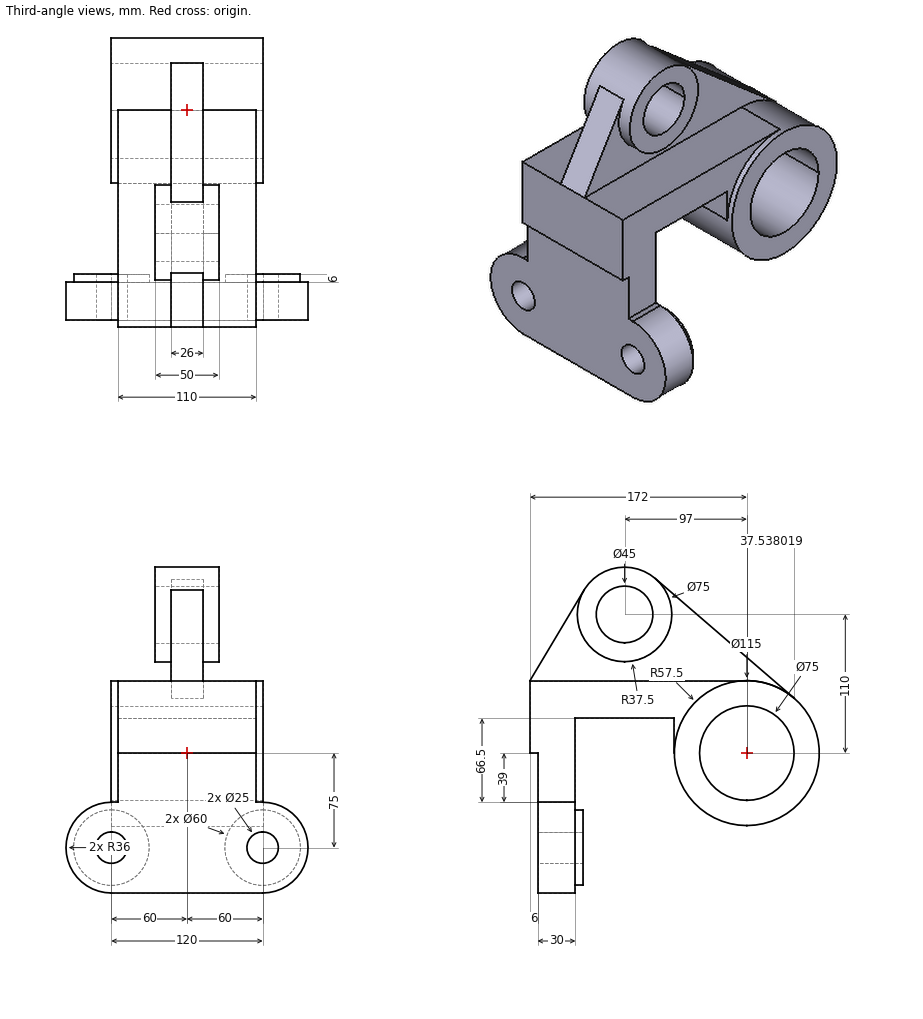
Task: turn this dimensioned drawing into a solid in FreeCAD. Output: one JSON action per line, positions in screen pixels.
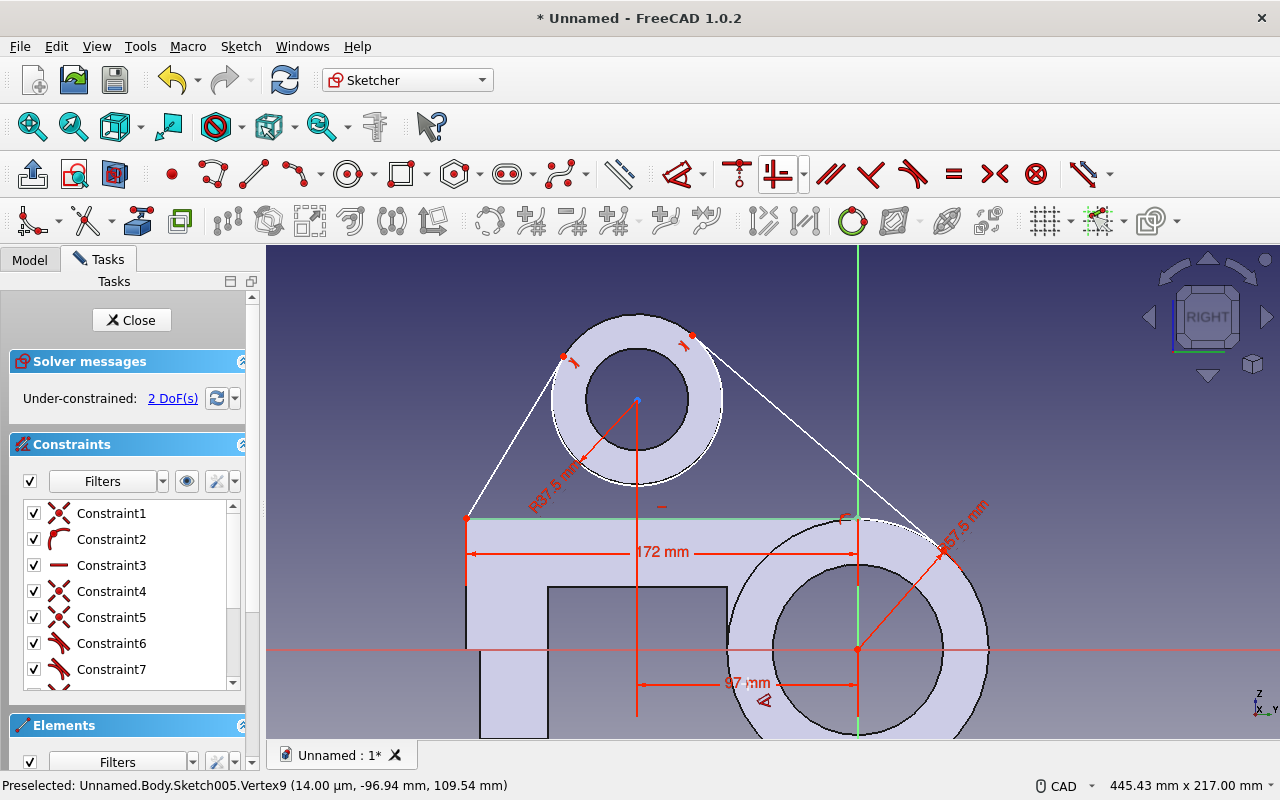
{"action": "left_click", "coordinate": [637, 400]}
{"action": "left_click", "coordinate": [892, 468]}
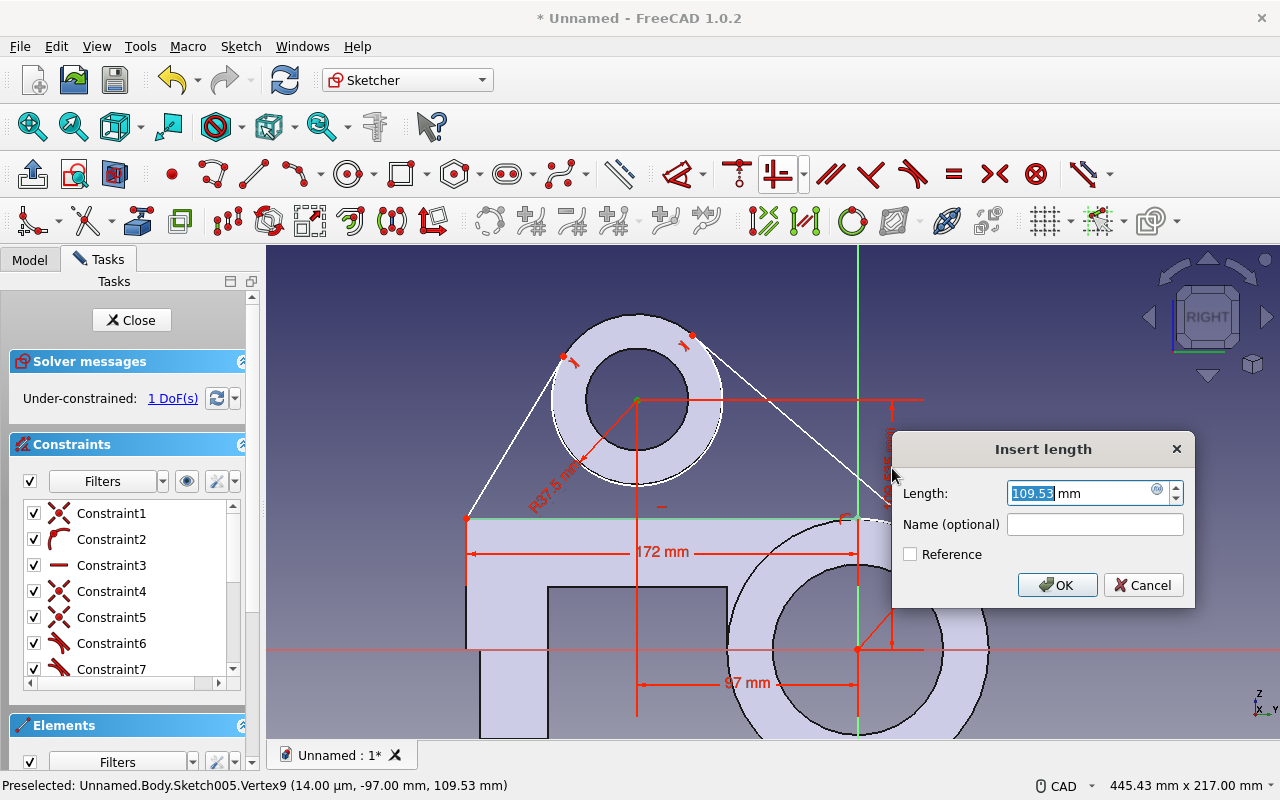
{"action": "type", "text": "110"}
{"action": "key", "text": "Return"}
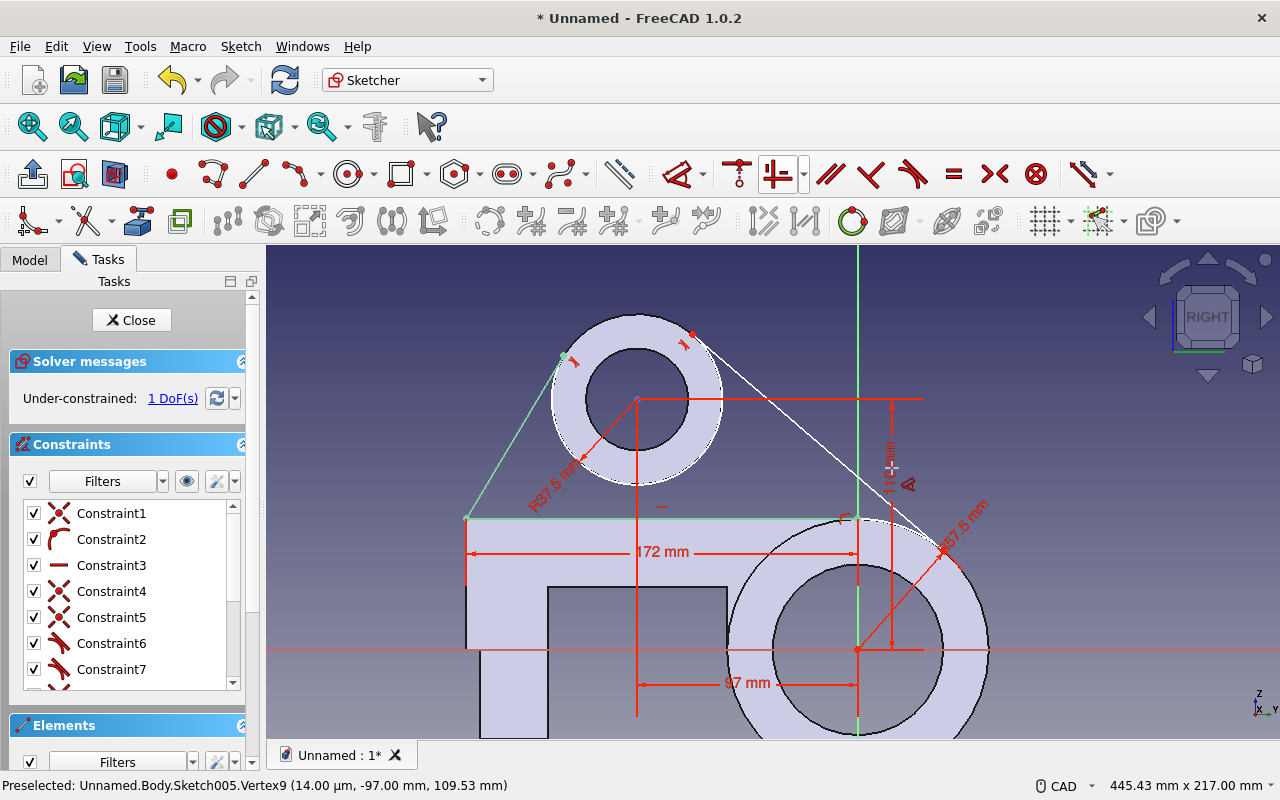
{"action": "left_click", "coordinate": [943, 550]}
{"action": "left_click", "coordinate": [901, 684]}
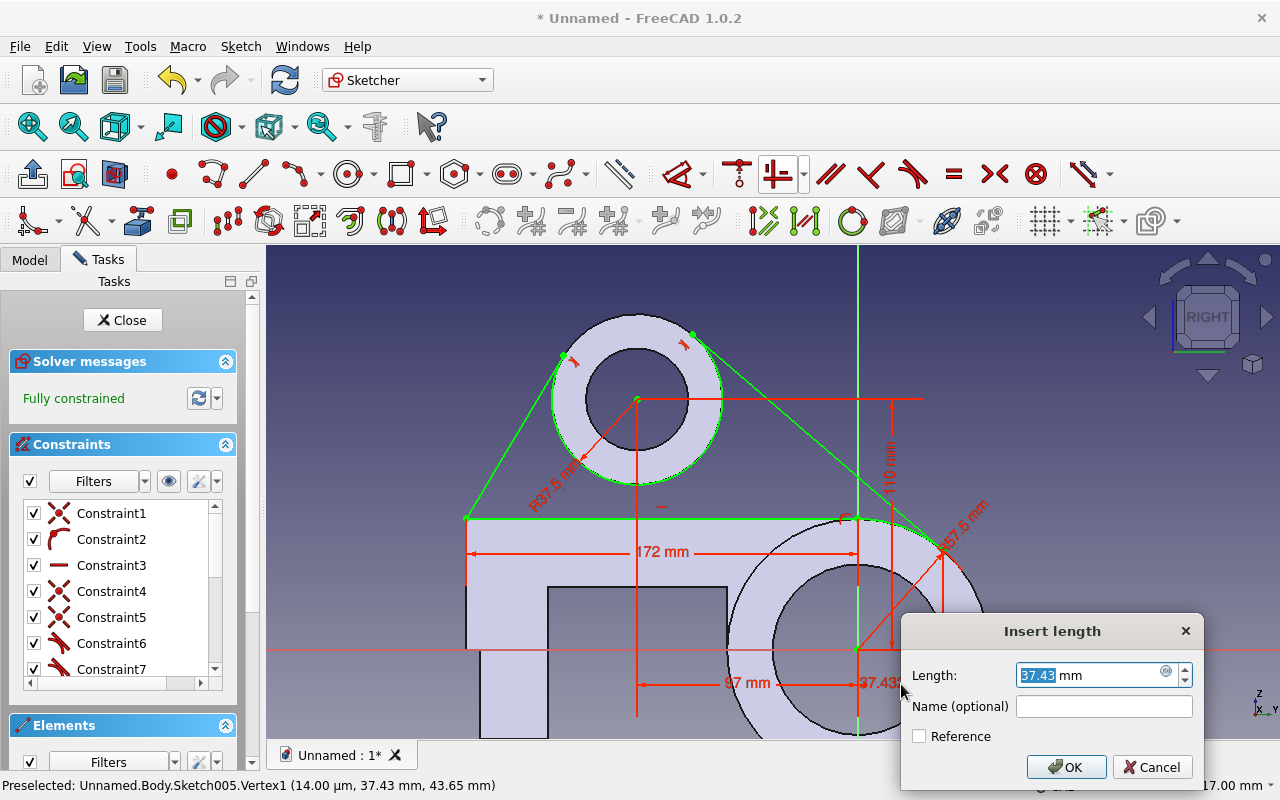
{"action": "type", "text": "37.538019"}
{"action": "key", "text": "Return"}
{"action": "key", "text": "Escape"}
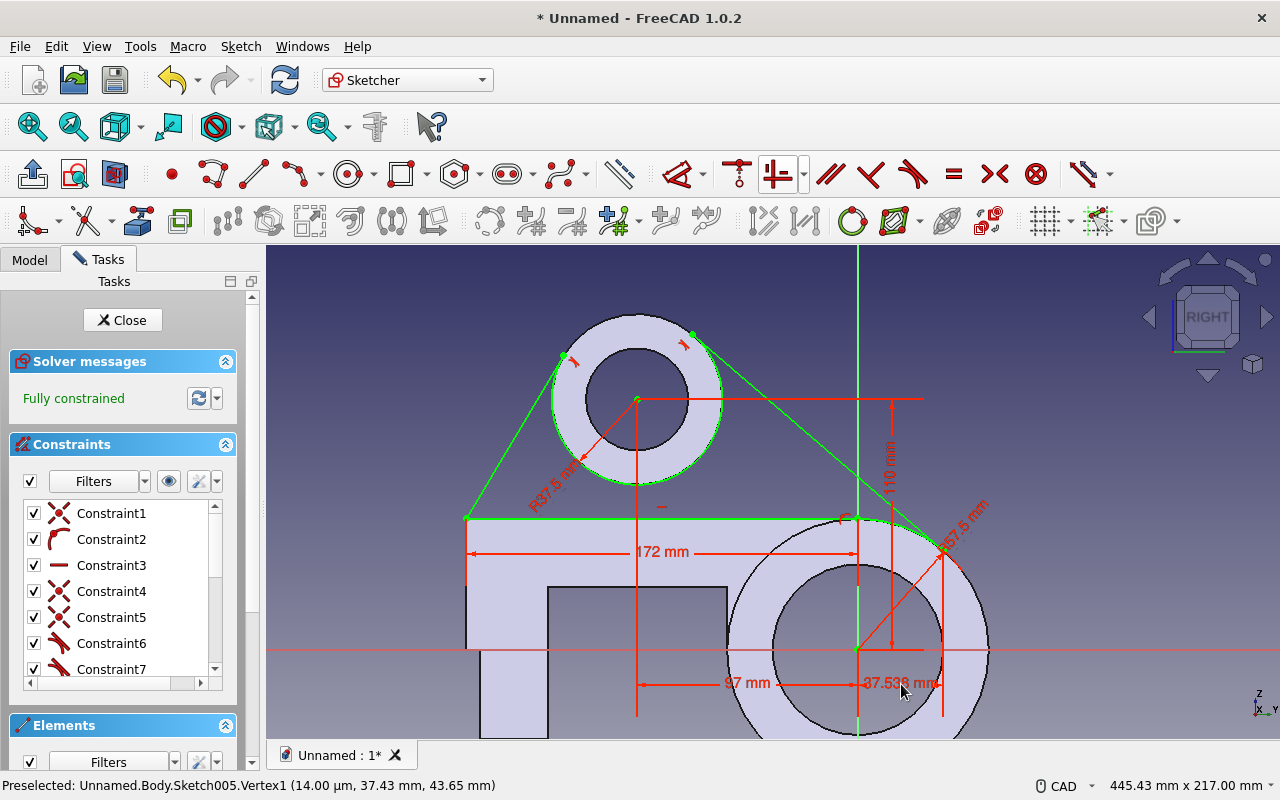
{"action": "left_click", "coordinate": [123, 320]}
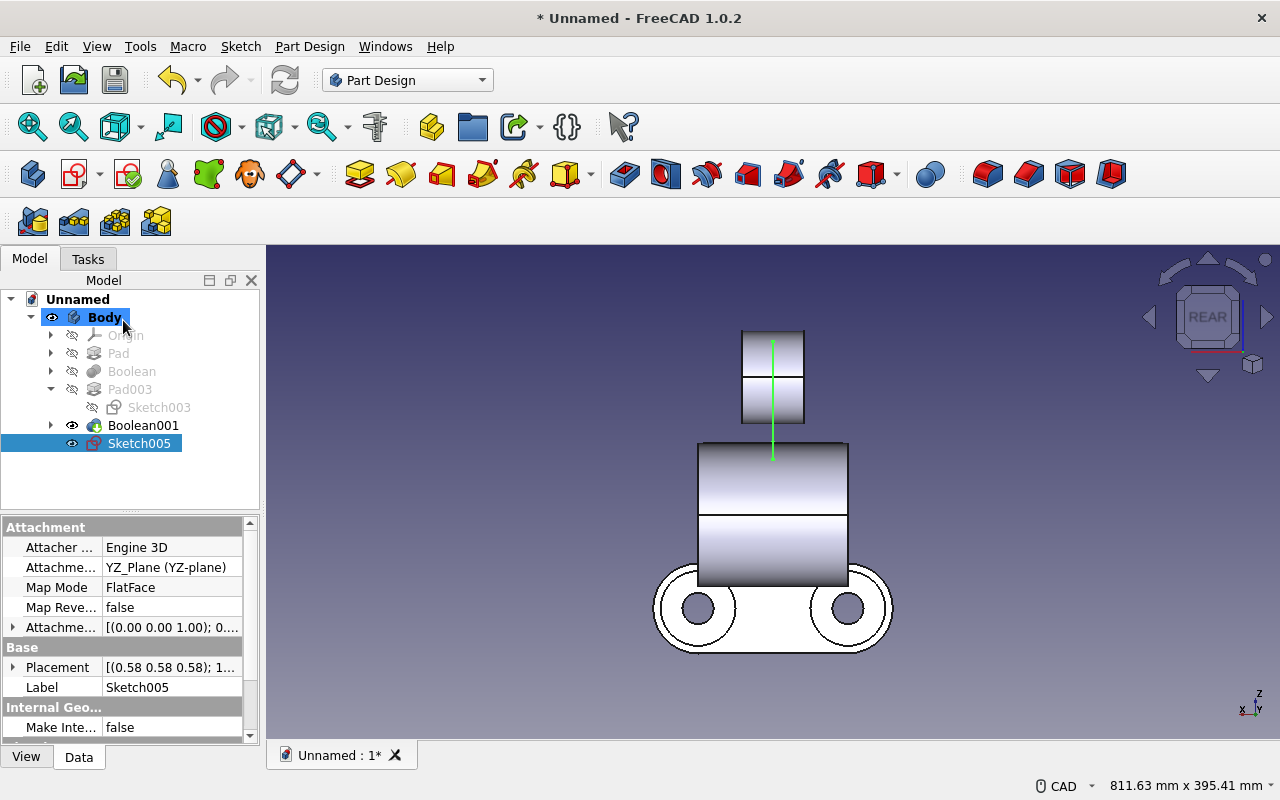
{"action": "left_click", "coordinate": [360, 174]}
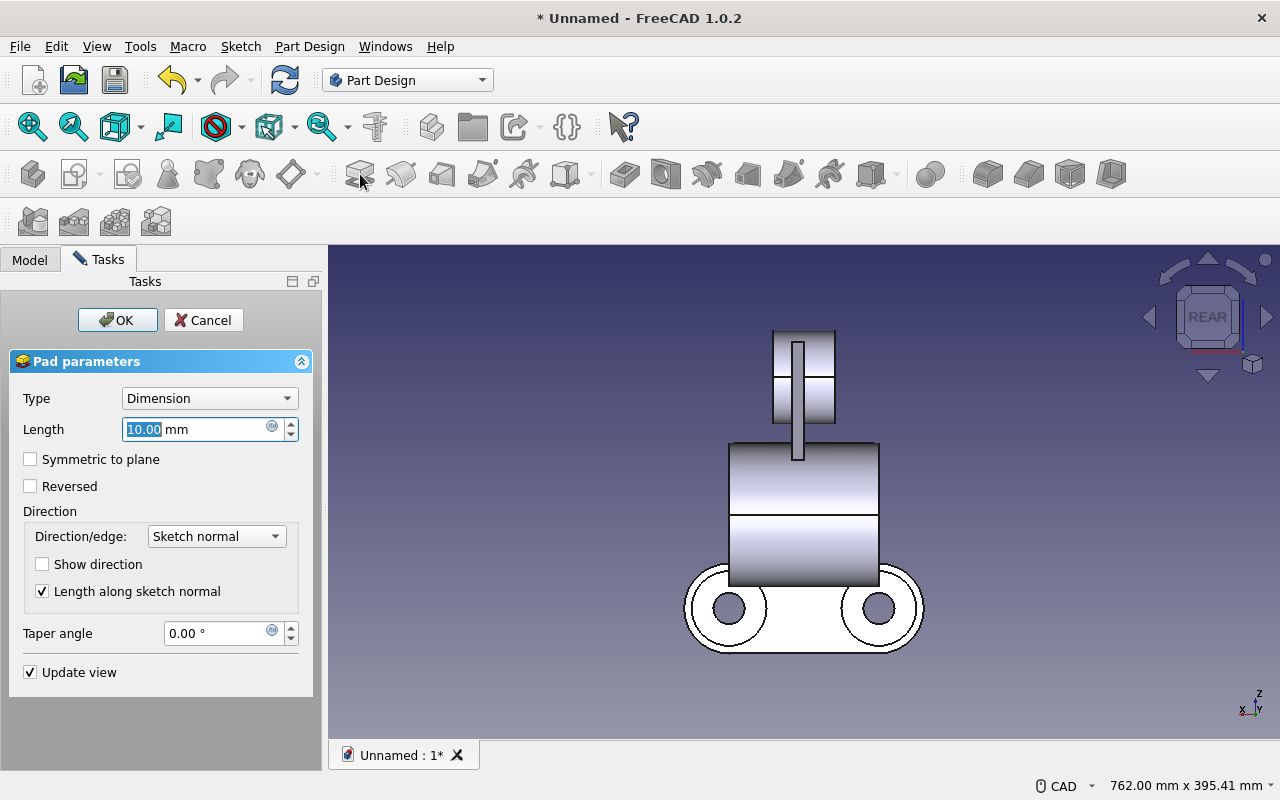
{"action": "type", "text": "26"}
{"action": "key", "text": "Tab"}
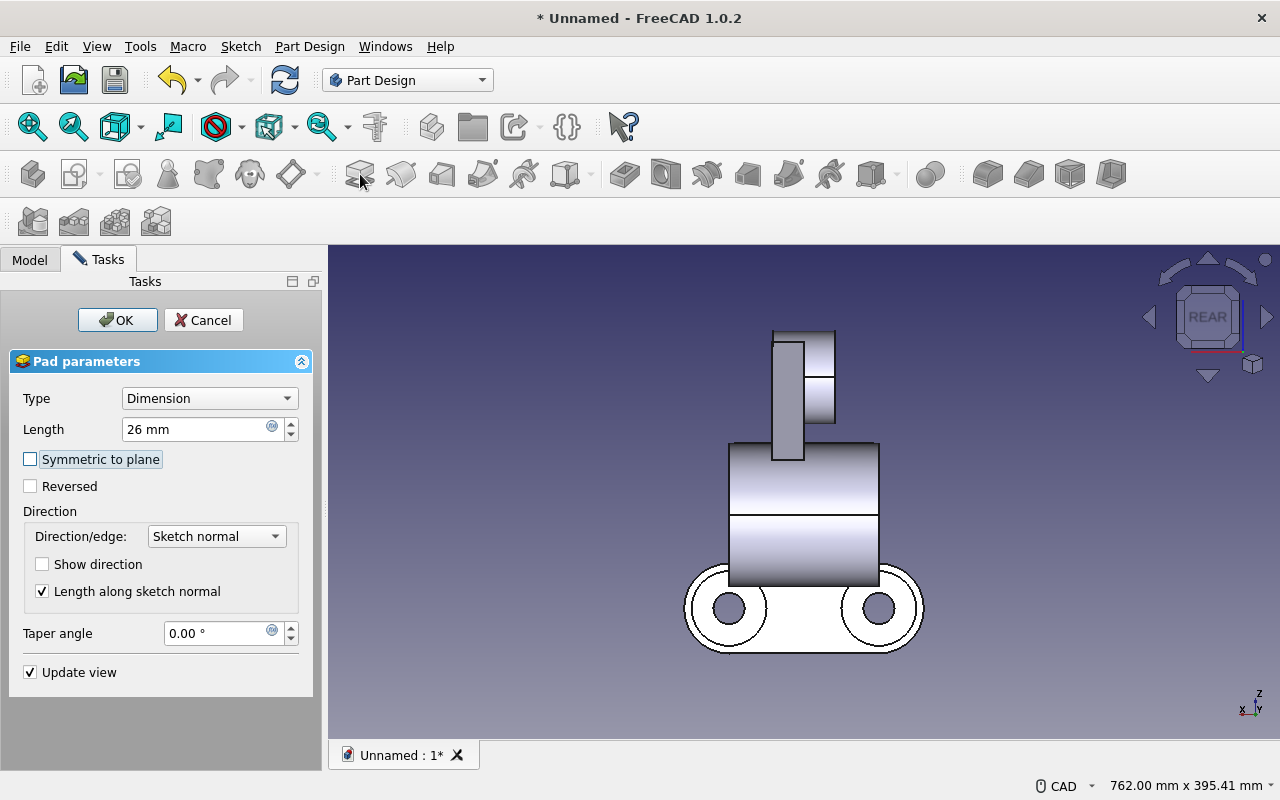
{"action": "left_click", "coordinate": [31, 459]}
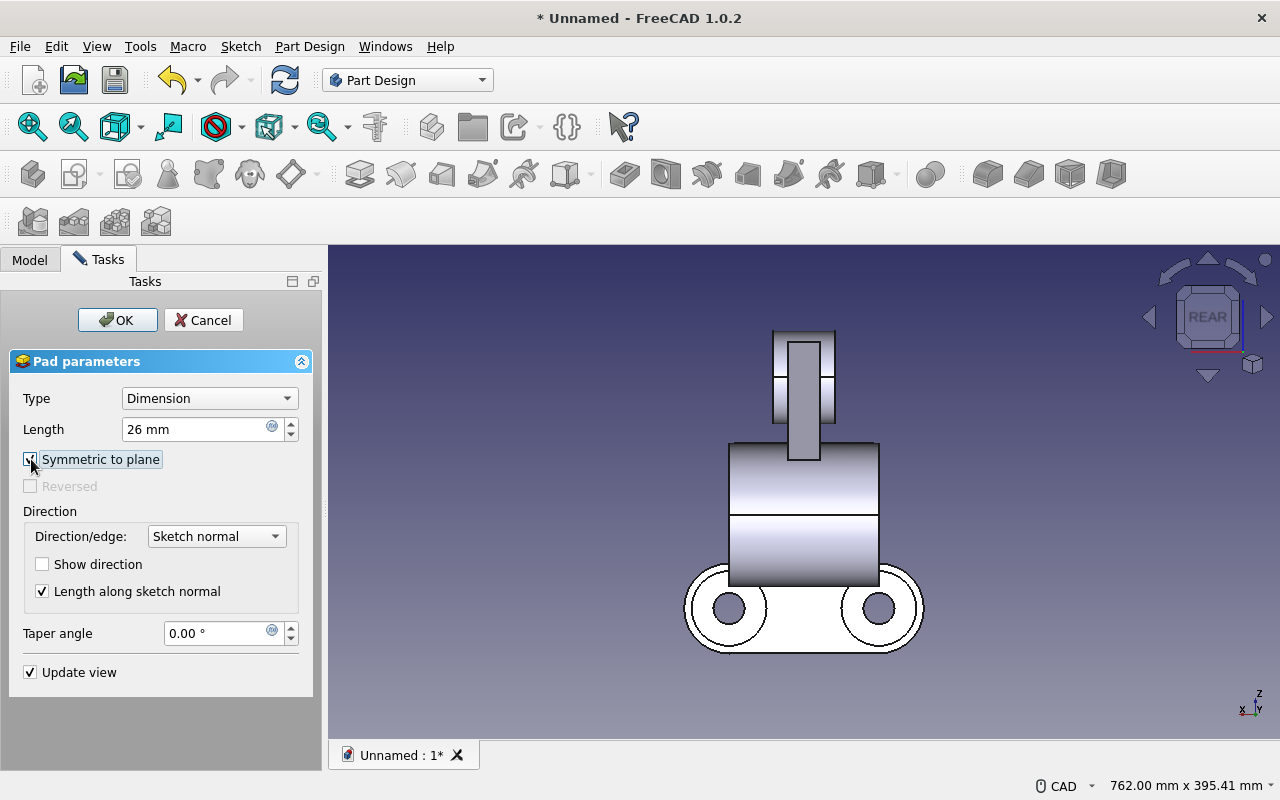
{"action": "left_click", "coordinate": [118, 320]}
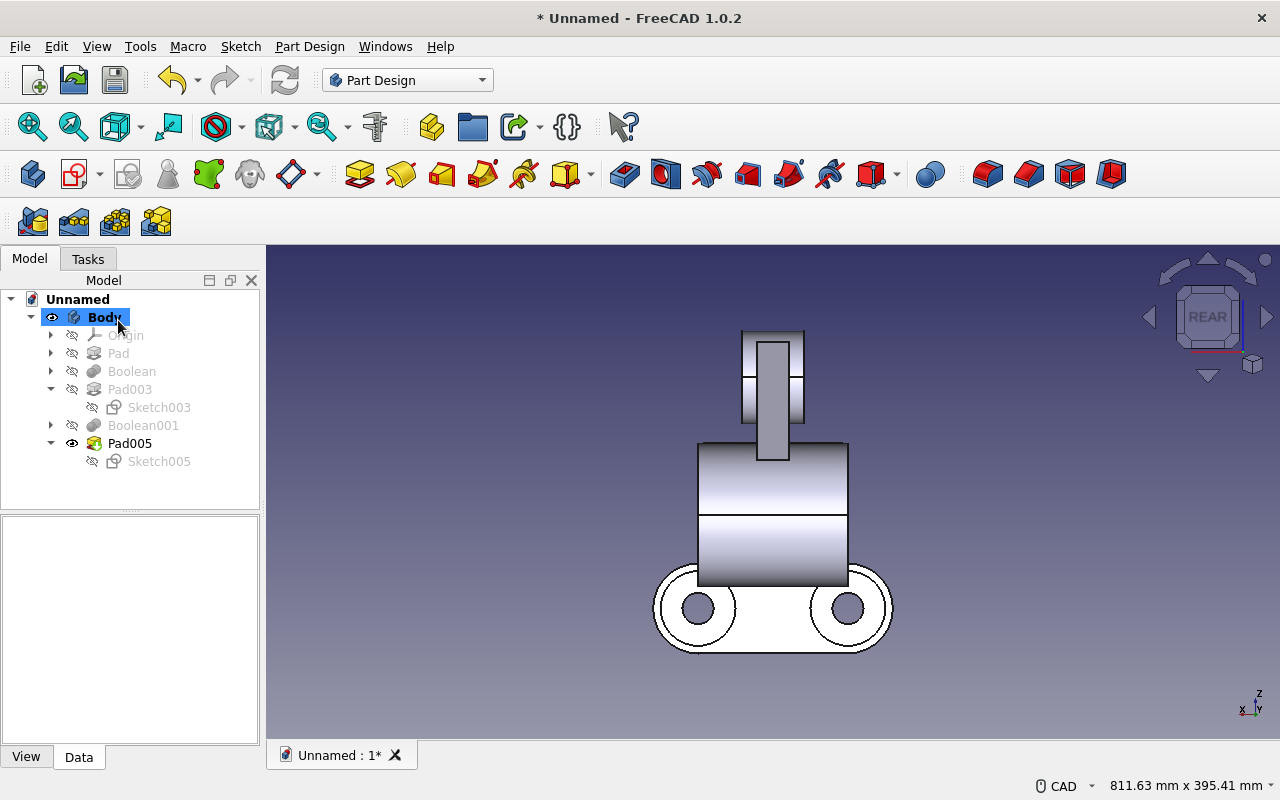
{"action": "key", "text": "0"}